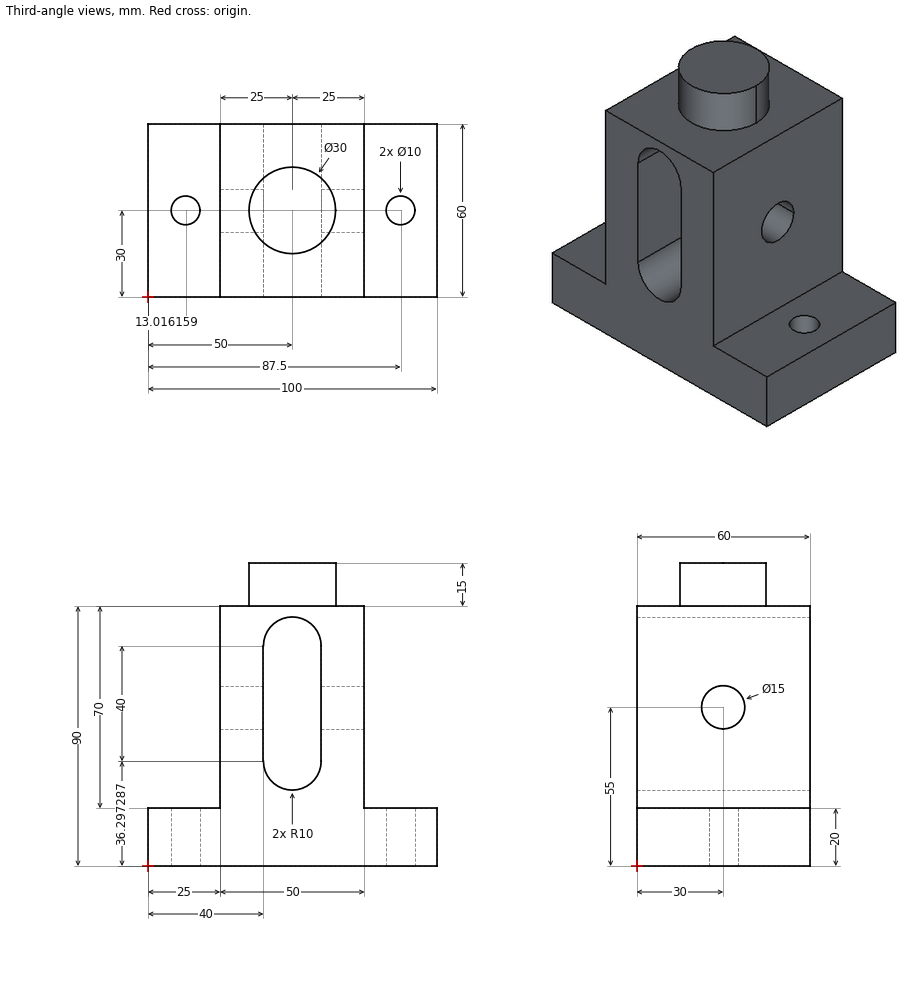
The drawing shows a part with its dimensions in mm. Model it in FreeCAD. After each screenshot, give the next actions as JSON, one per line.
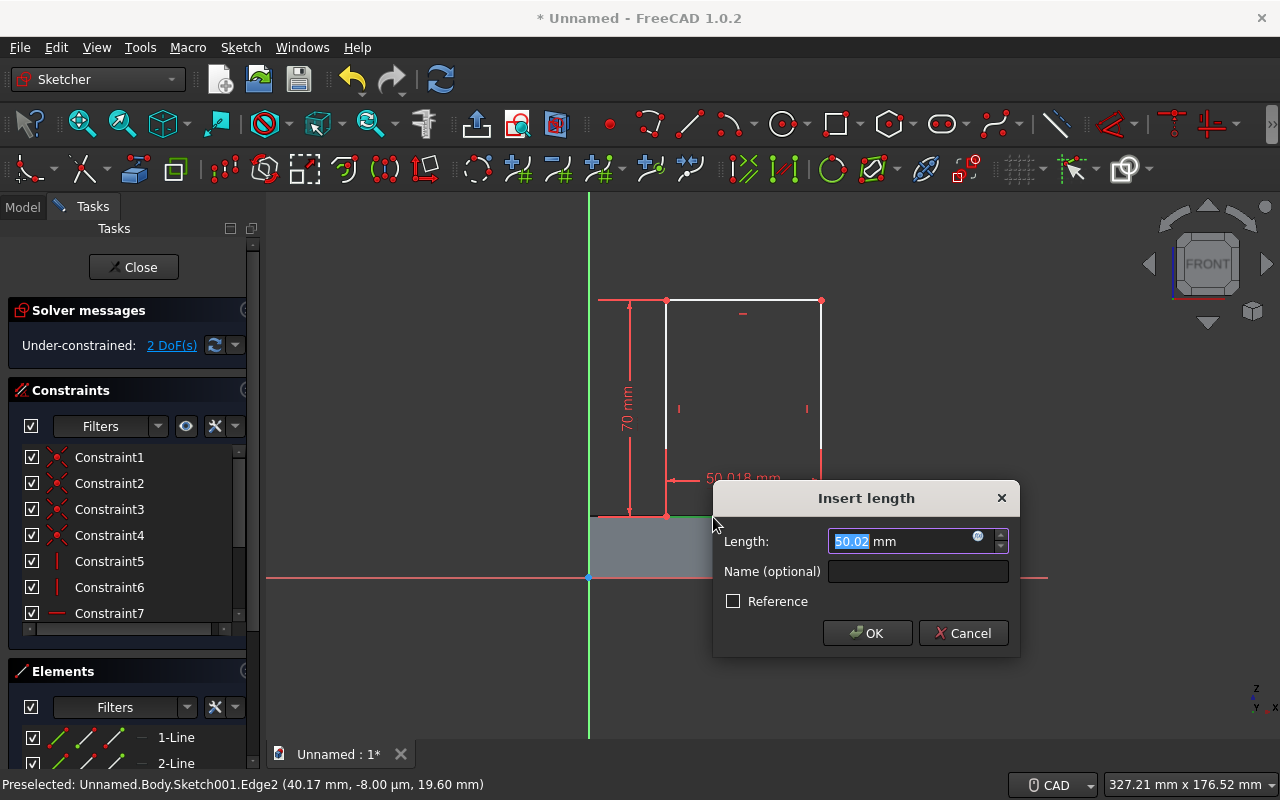
{"action": "type", "text": "50"}
{"action": "key", "text": "Return"}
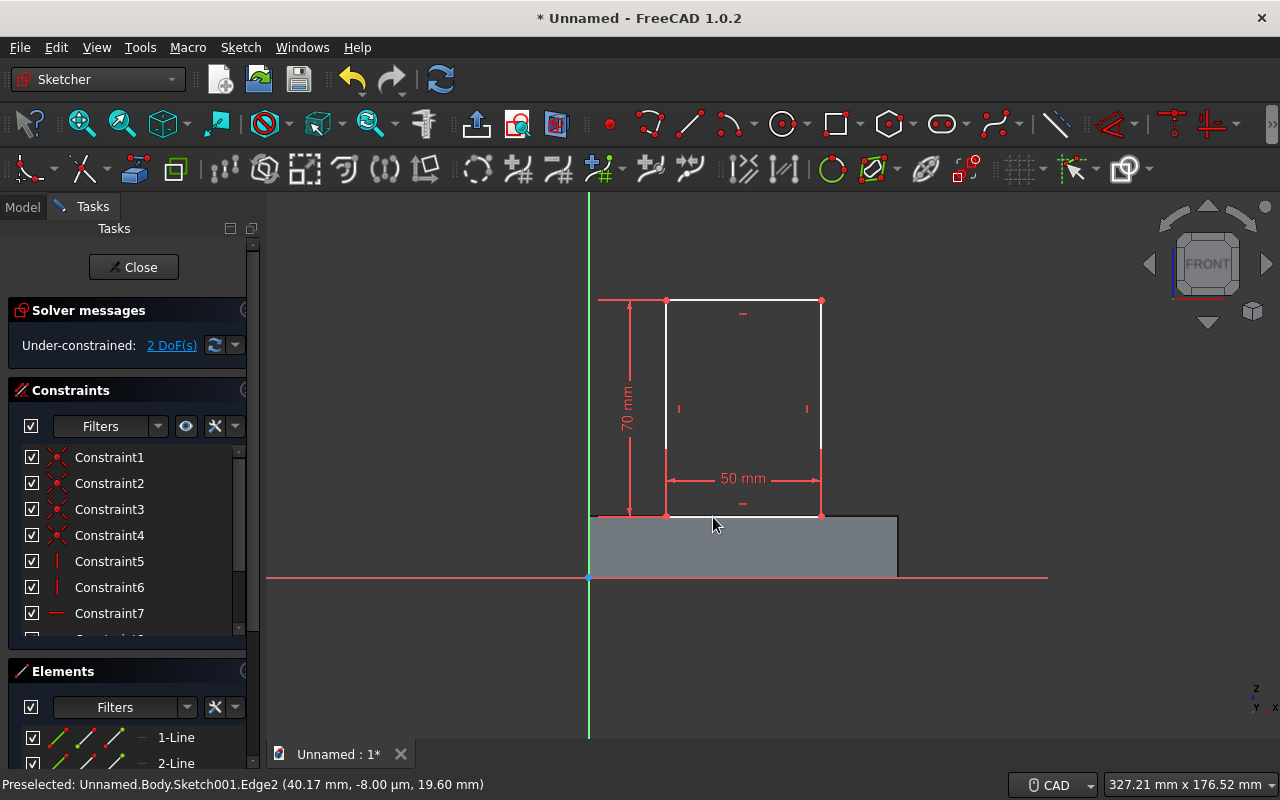
{"action": "left_click", "coordinate": [666, 300]}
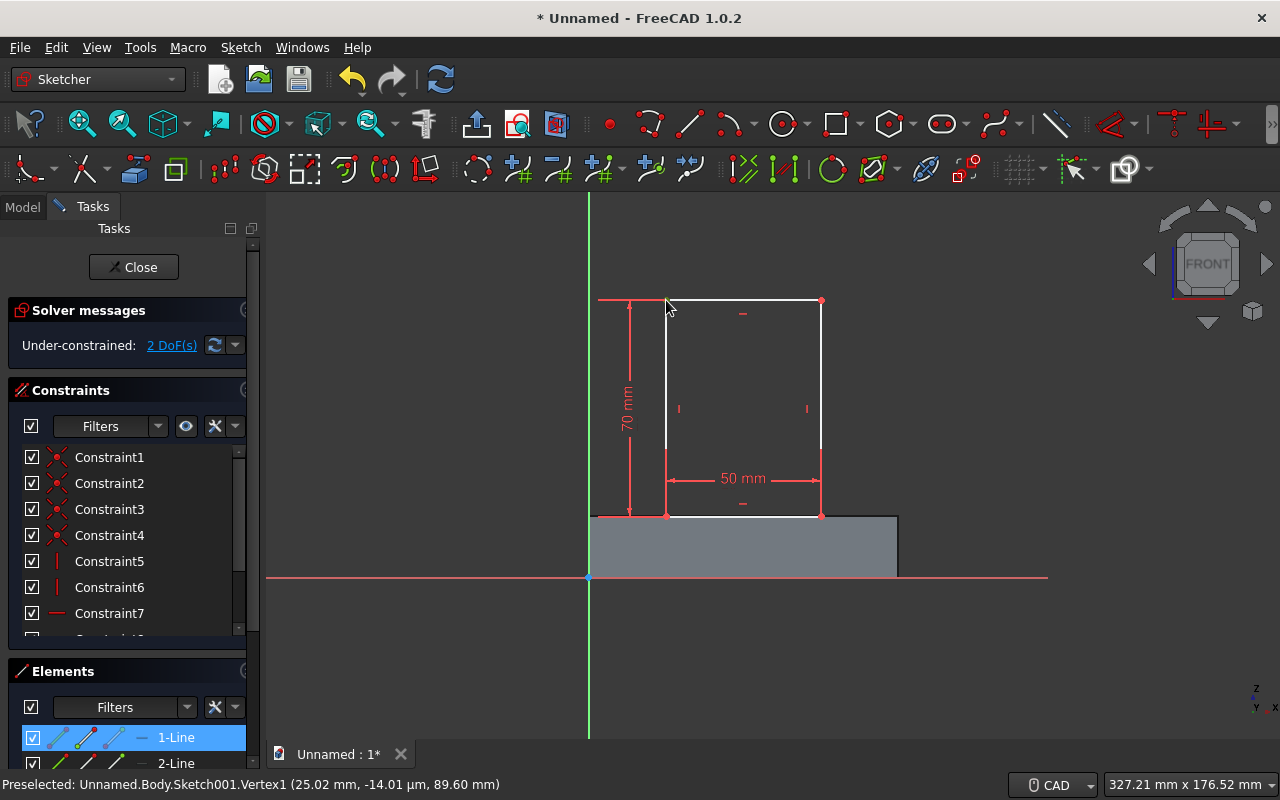
{"action": "key", "text": "l"}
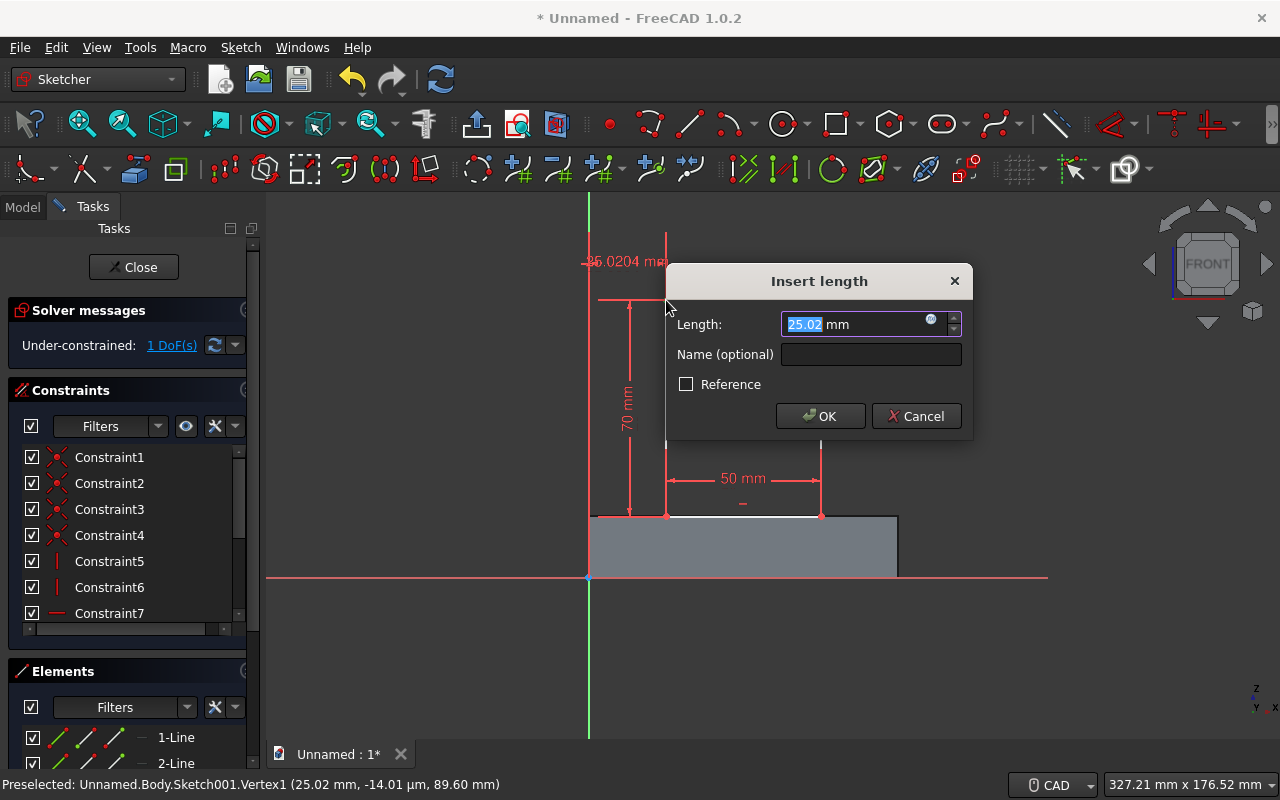
{"action": "type", "text": "25"}
{"action": "key", "text": "Return"}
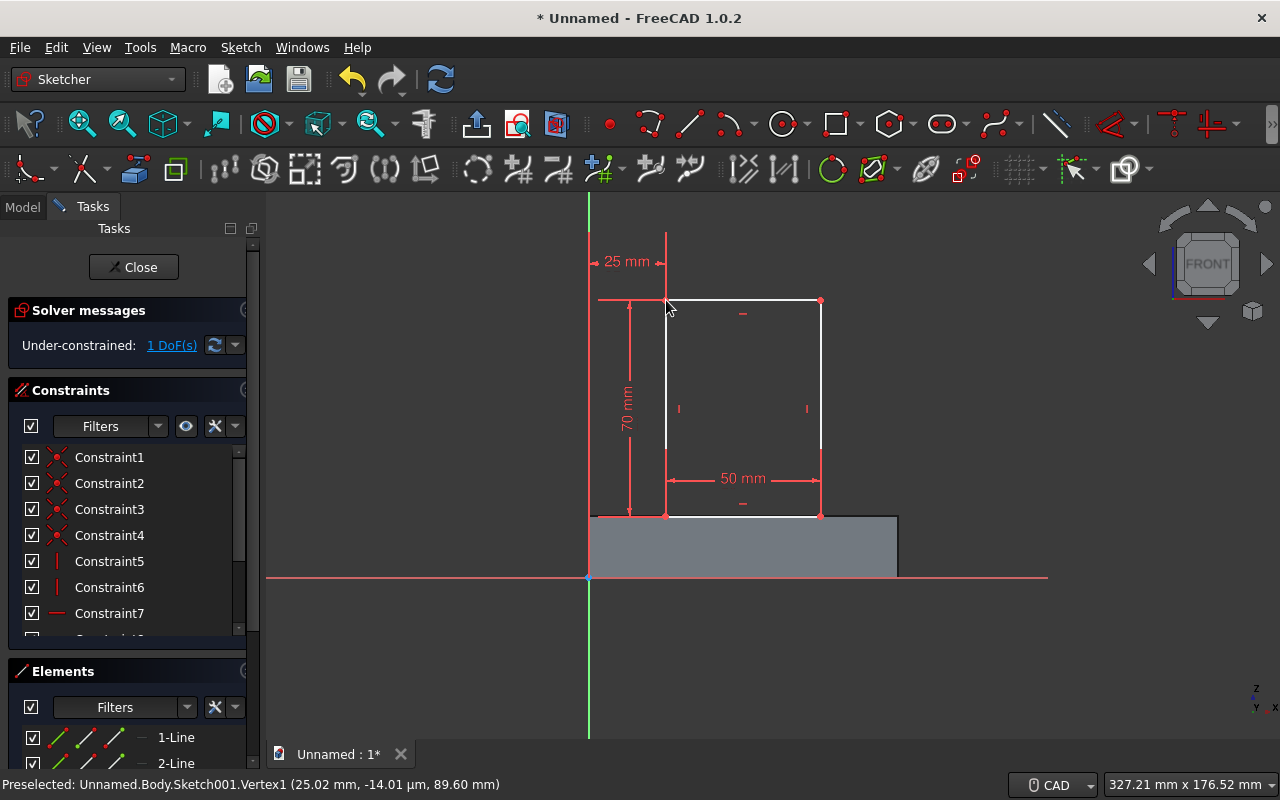
{"action": "left_click", "coordinate": [666, 300]}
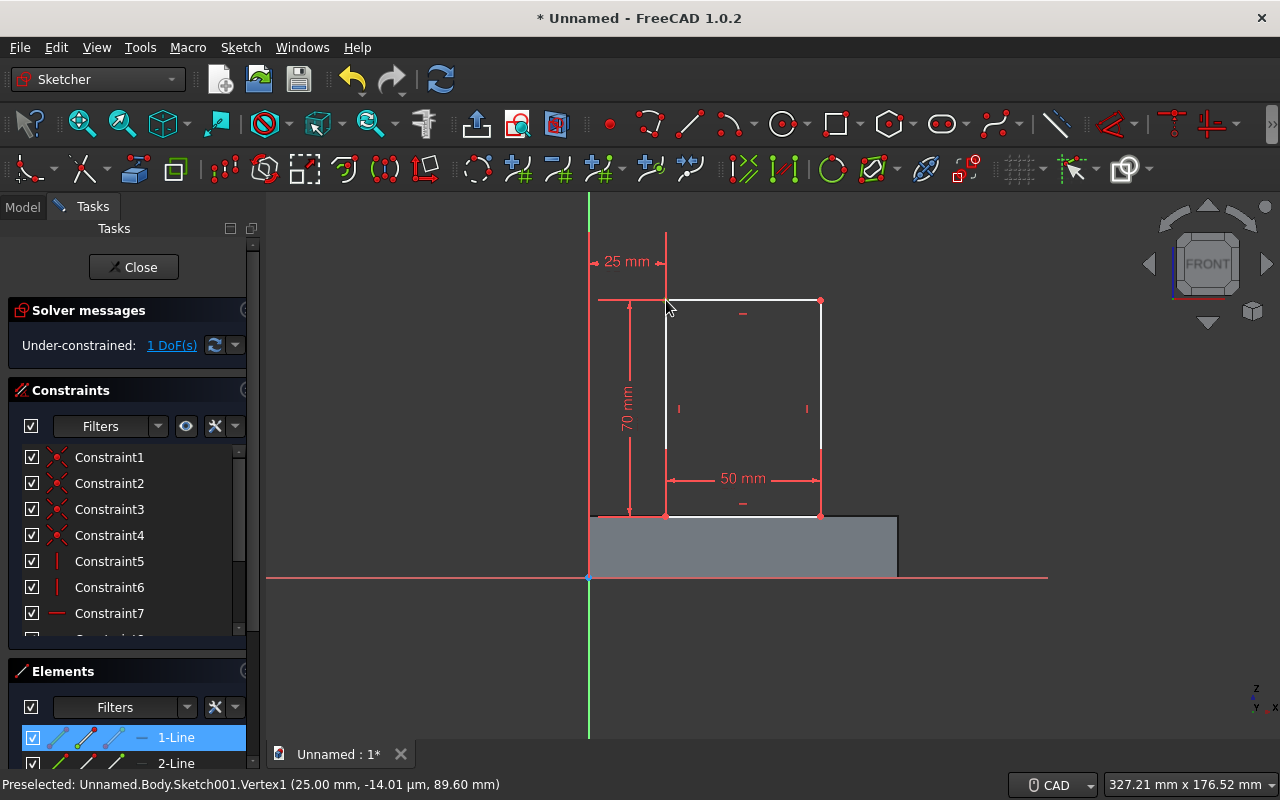
{"action": "key", "text": "i"}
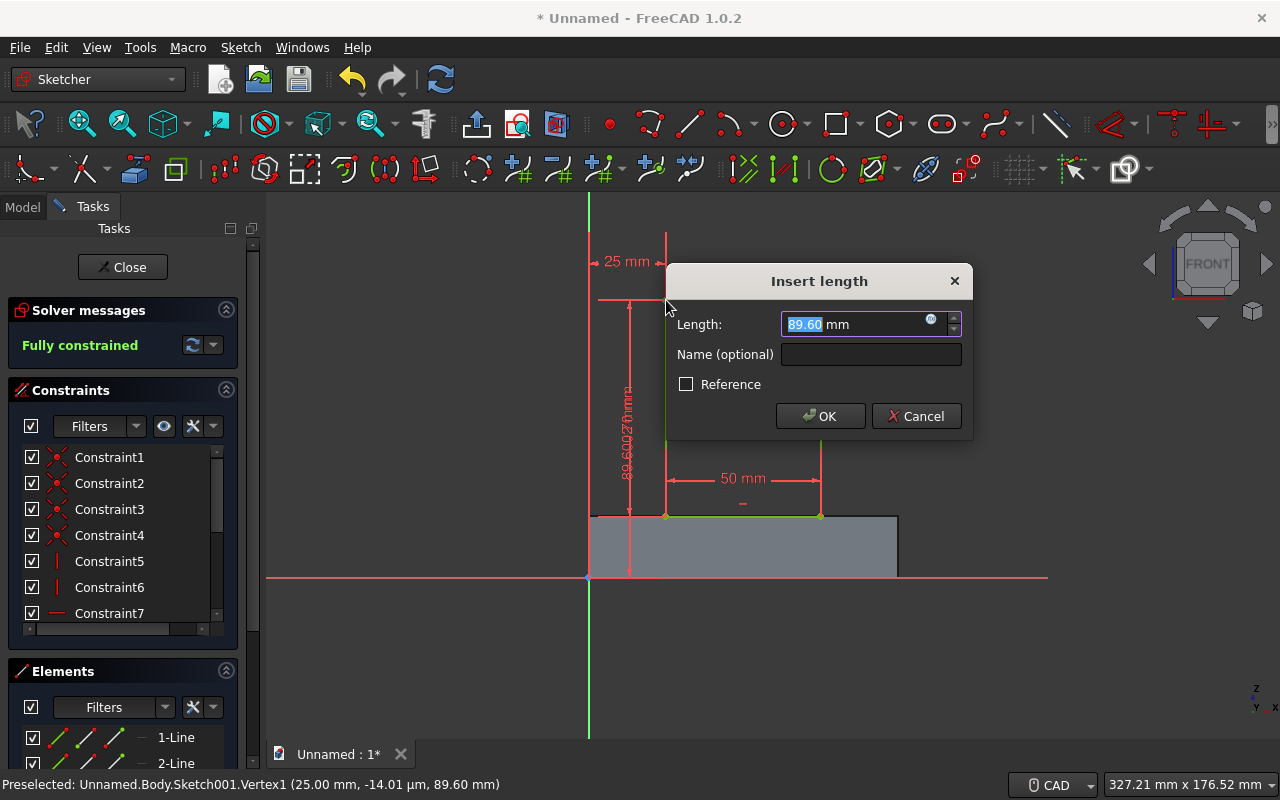
{"action": "type", "text": "90"}
{"action": "key", "text": "Return"}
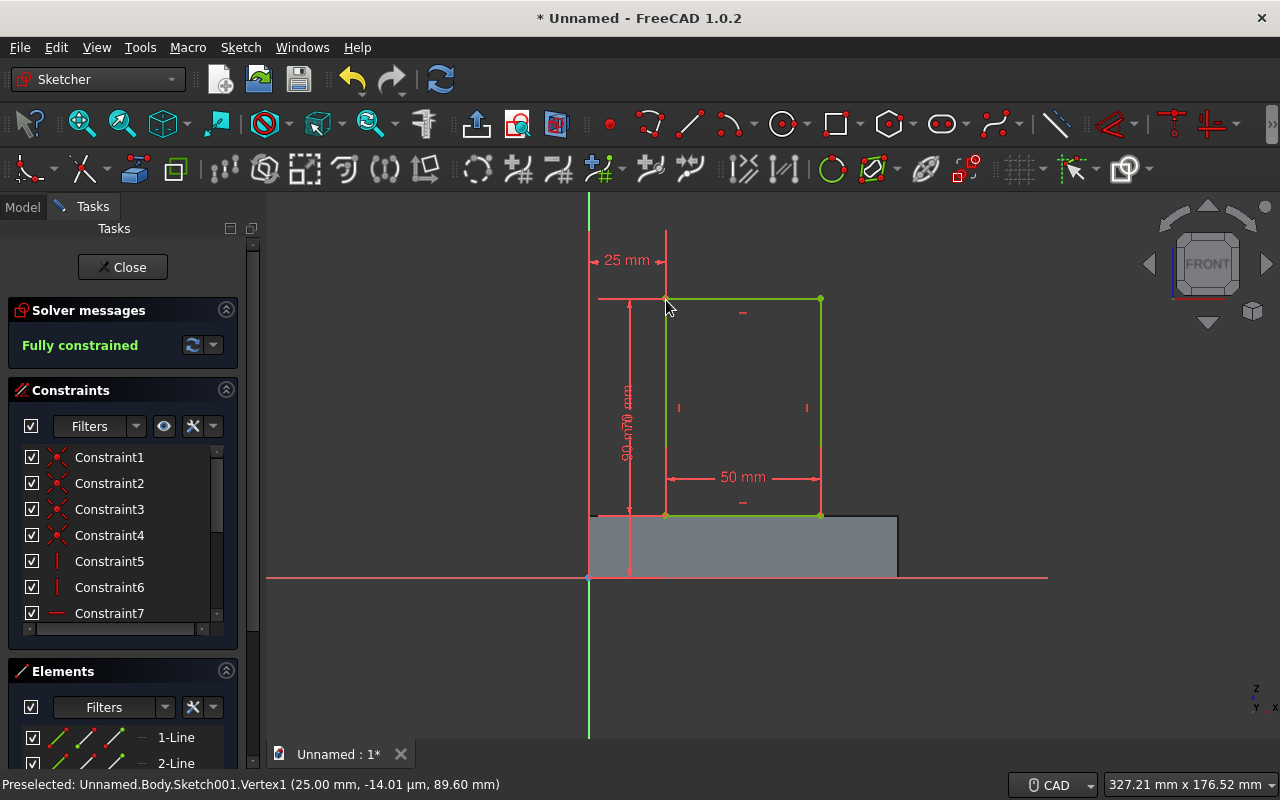
{"action": "left_click", "coordinate": [123, 267]}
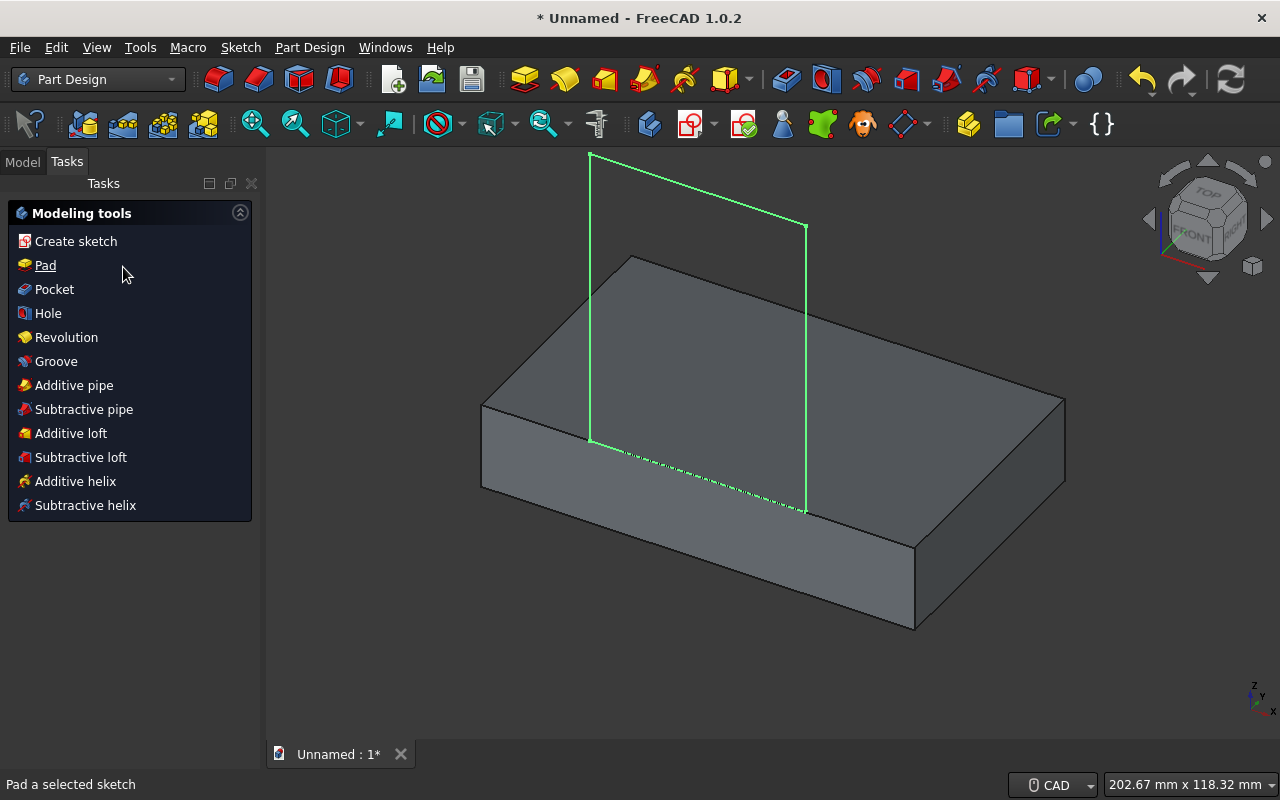
{"action": "left_click", "coordinate": [526, 80]}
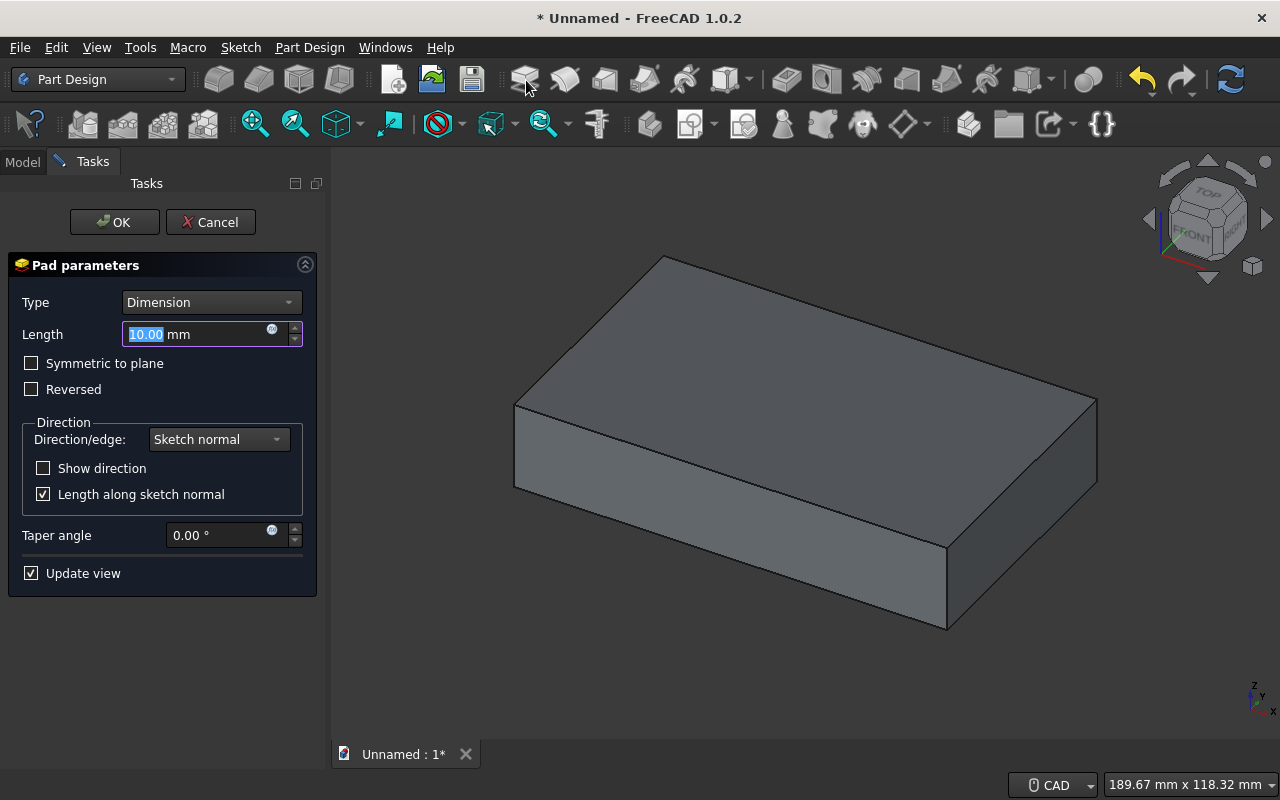
{"action": "type", "text": "60"}
{"action": "key", "text": "Tab"}